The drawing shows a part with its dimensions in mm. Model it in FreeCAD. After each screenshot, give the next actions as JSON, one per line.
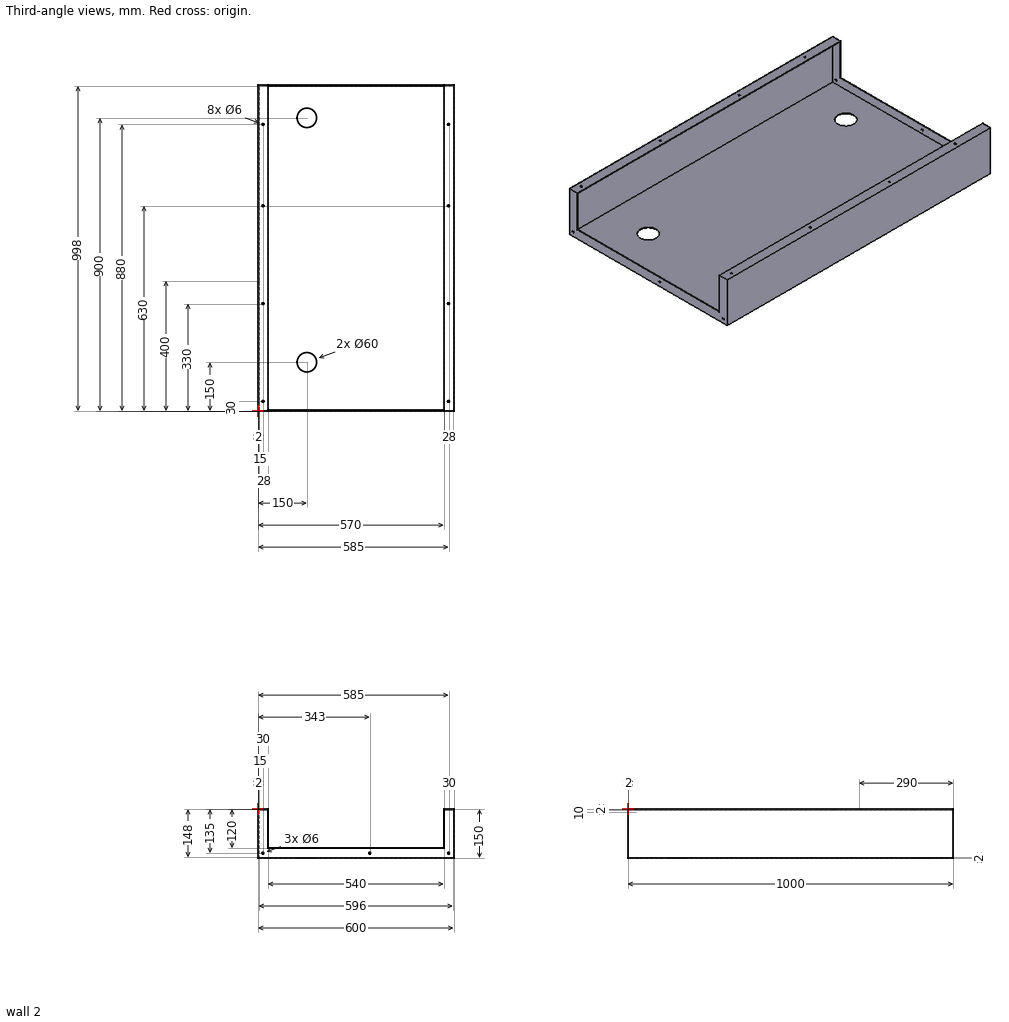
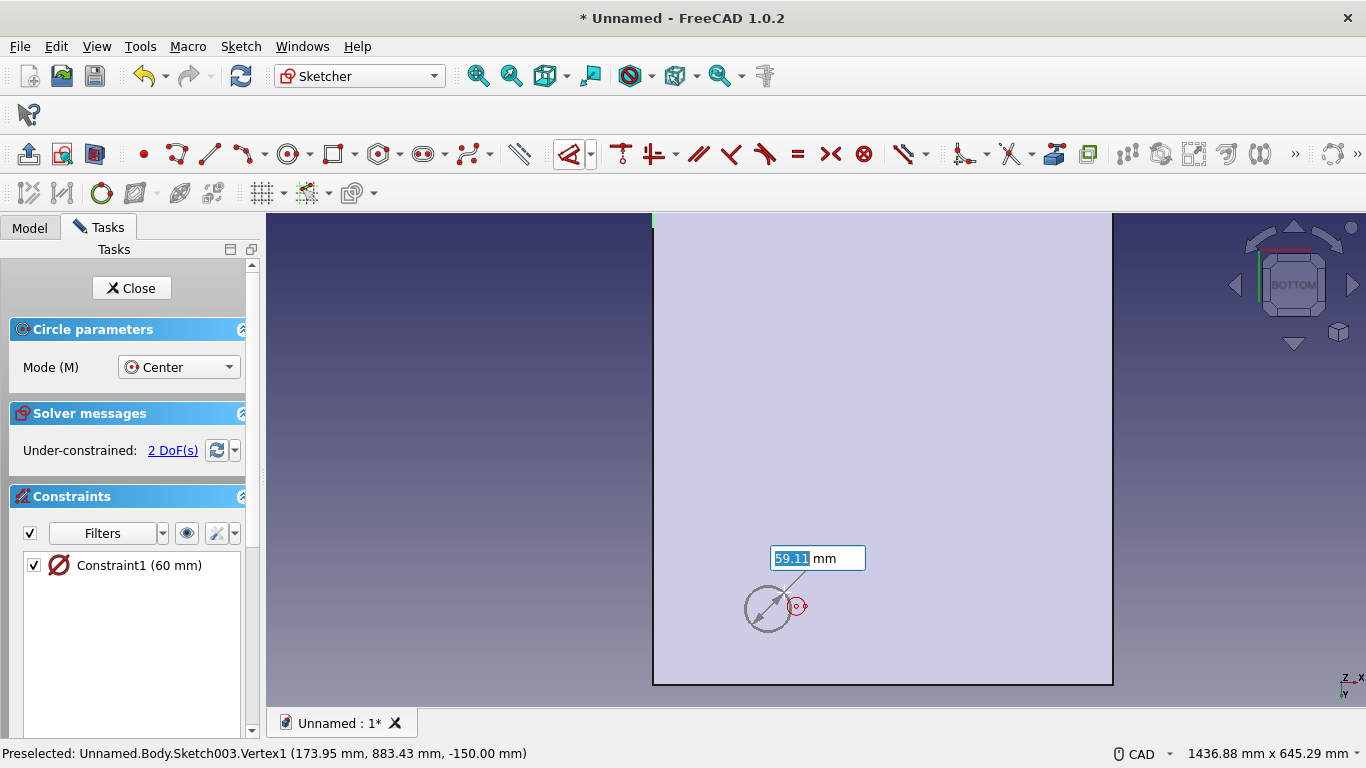
{"action": "type", "text": "60"}
{"action": "key", "text": "Return"}
{"action": "key", "text": "Escape"}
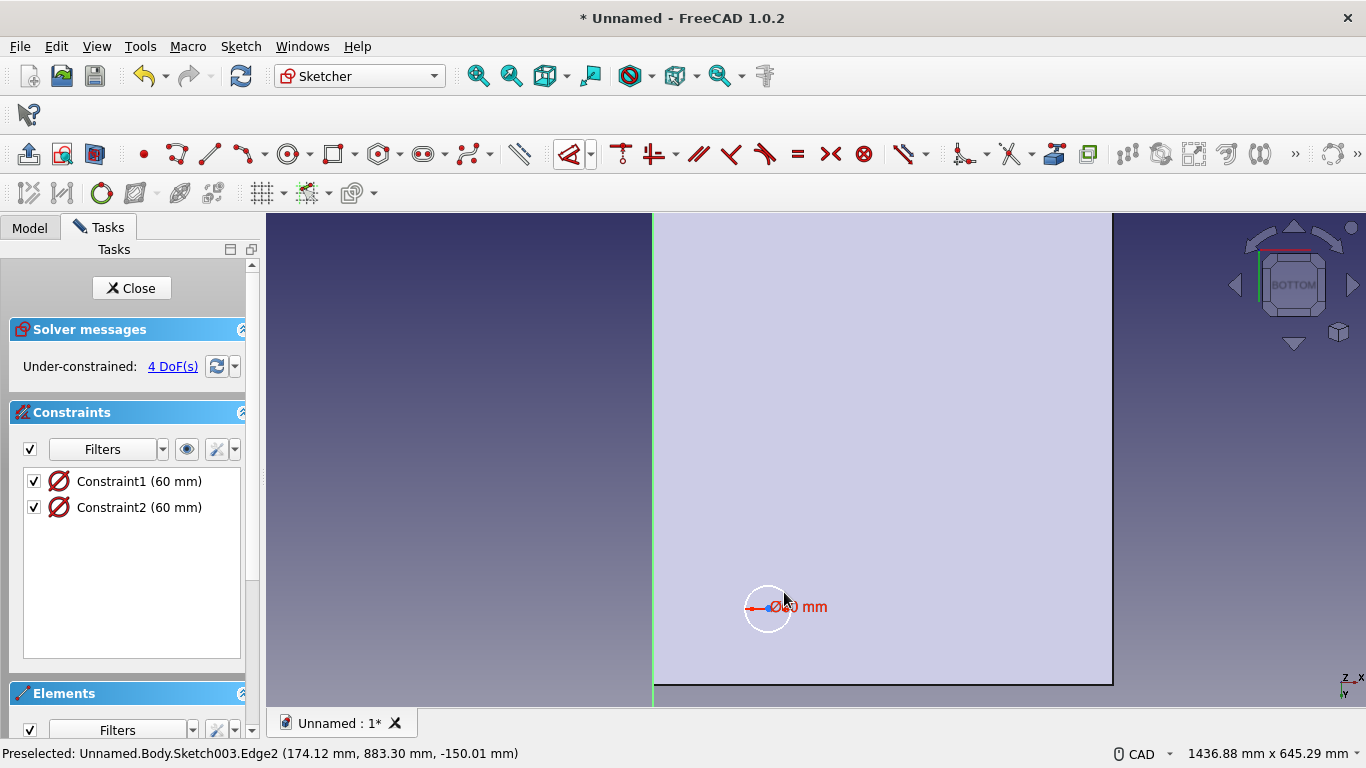
{"action": "scroll", "coordinate": [768, 611], "scroll_direction": "down", "scroll_amount": 4}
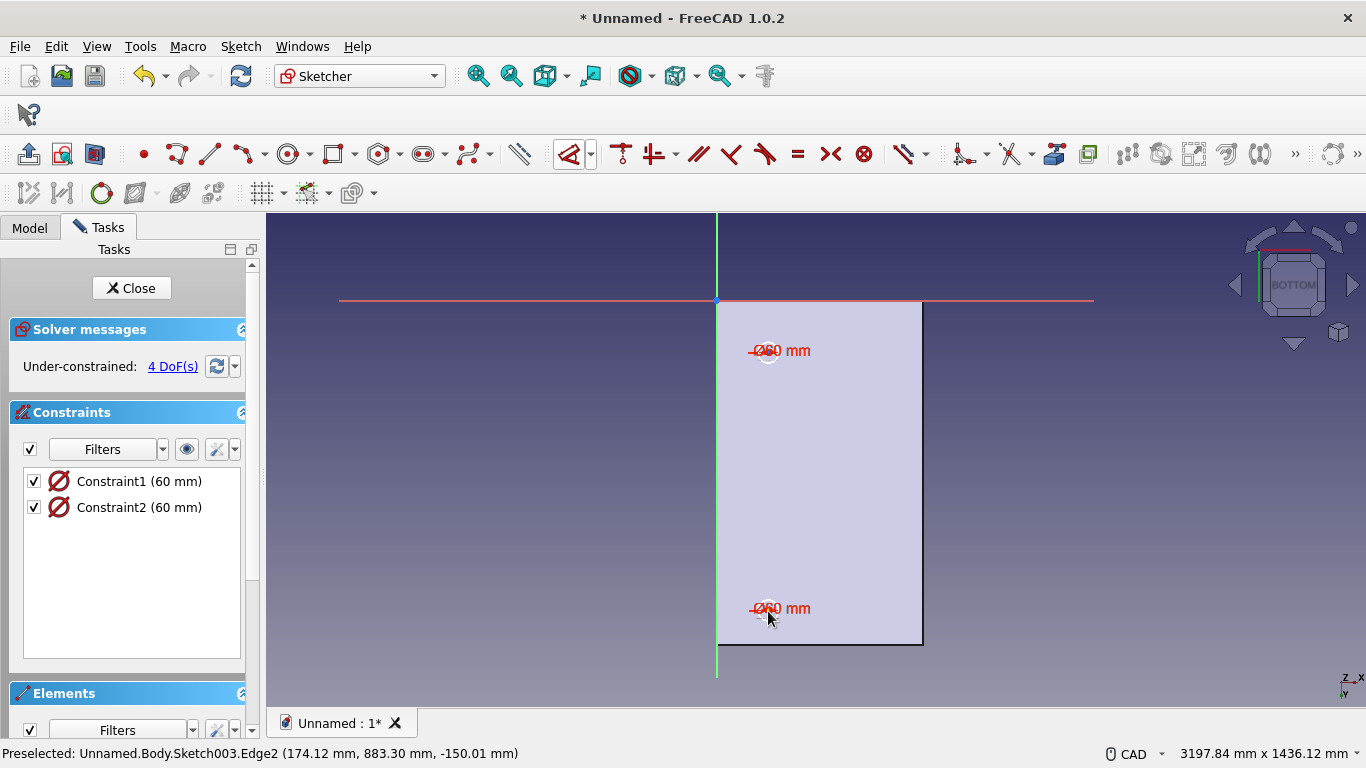
{"action": "left_click", "coordinate": [768, 353]}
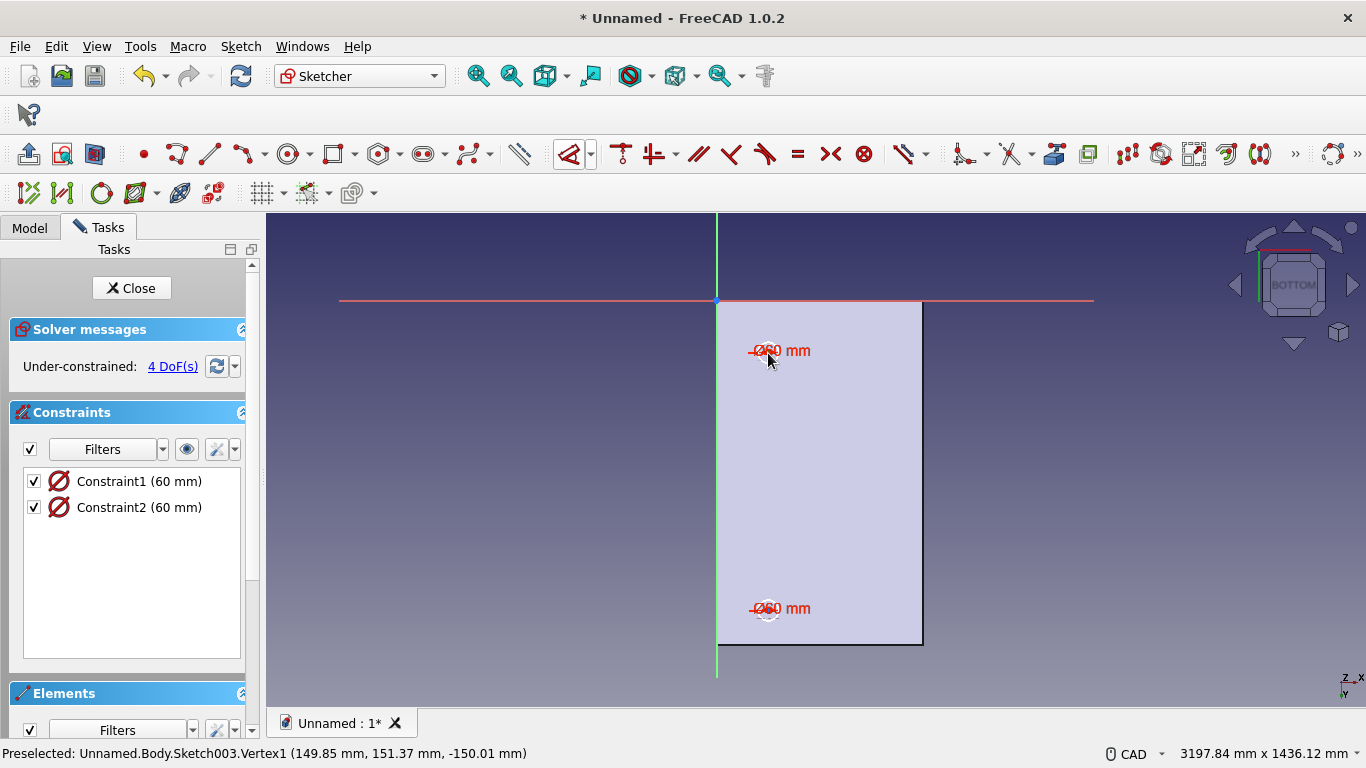
{"action": "left_click", "coordinate": [590, 154]}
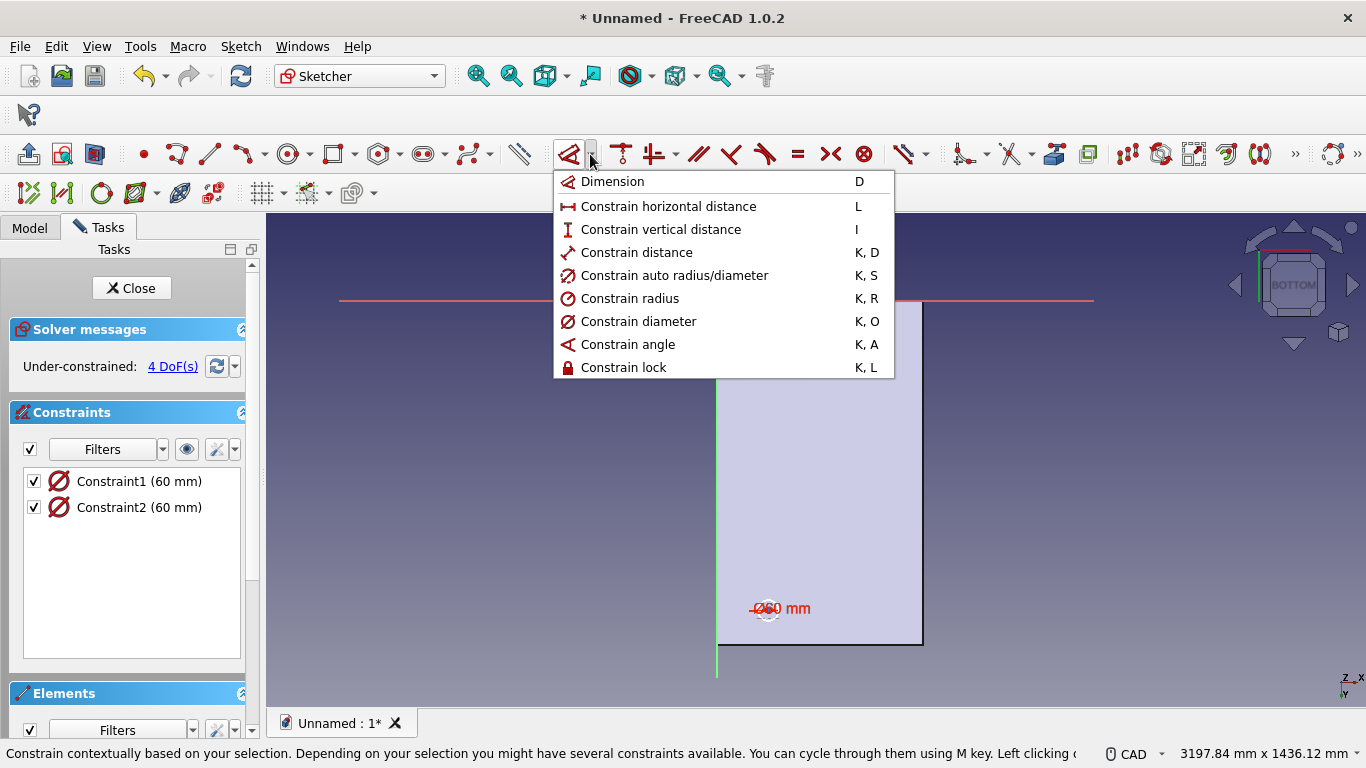
{"action": "left_click", "coordinate": [724, 206]}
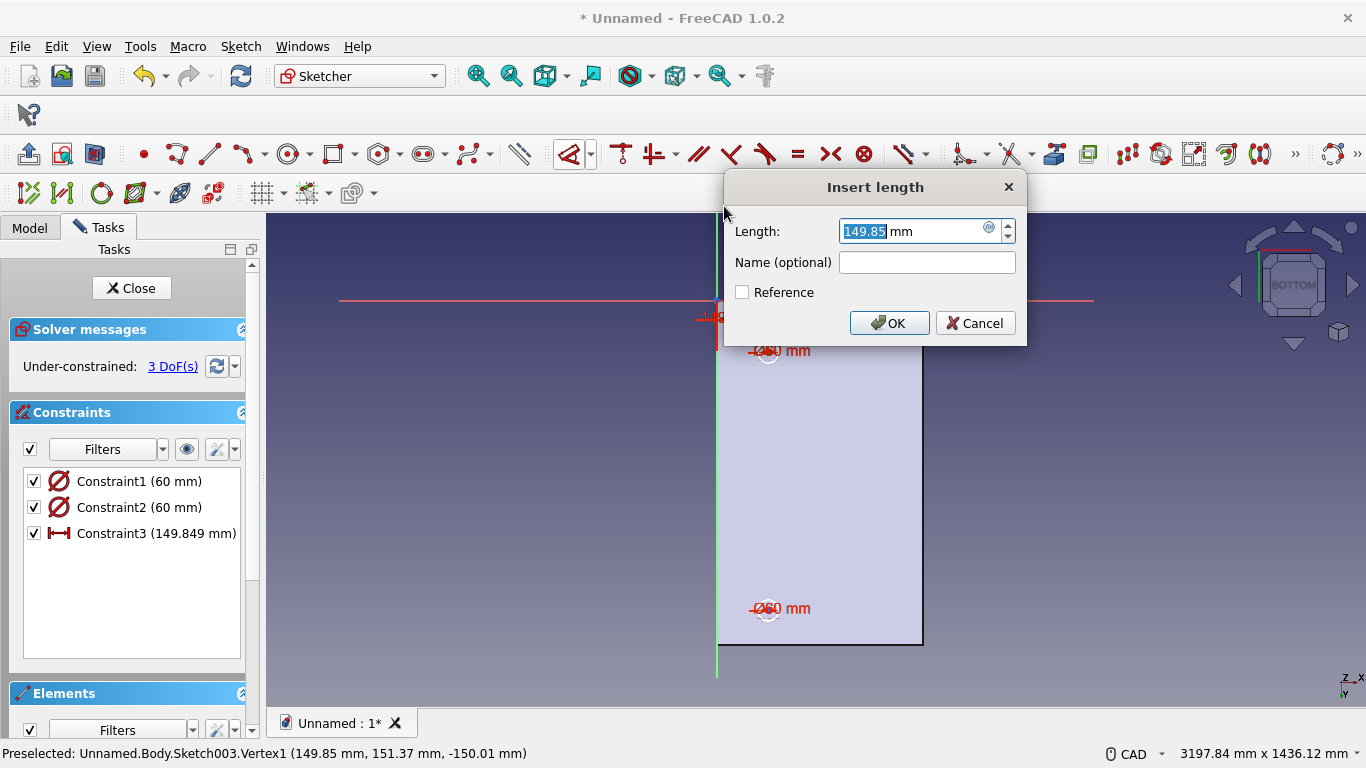
{"action": "type", "text": "150"}
{"action": "key", "text": "Return"}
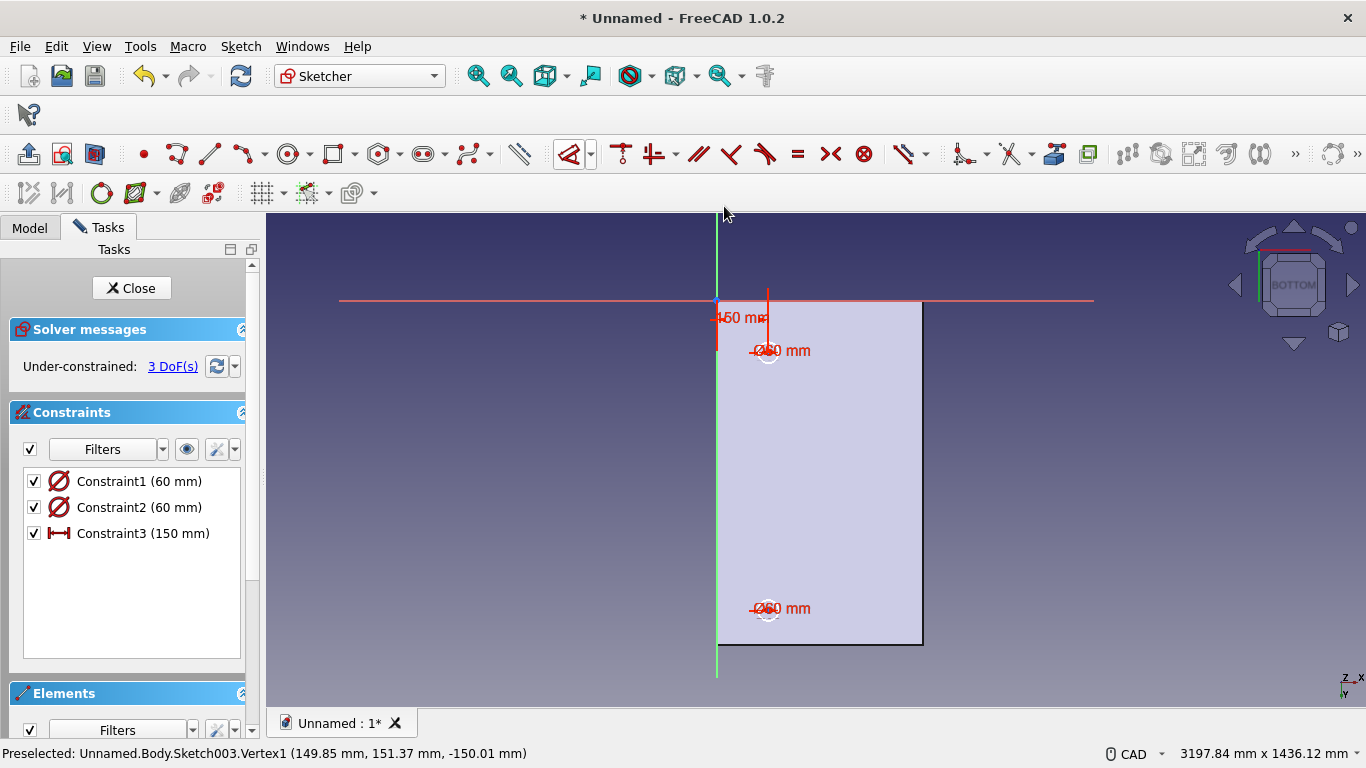
{"action": "left_click", "coordinate": [768, 353]}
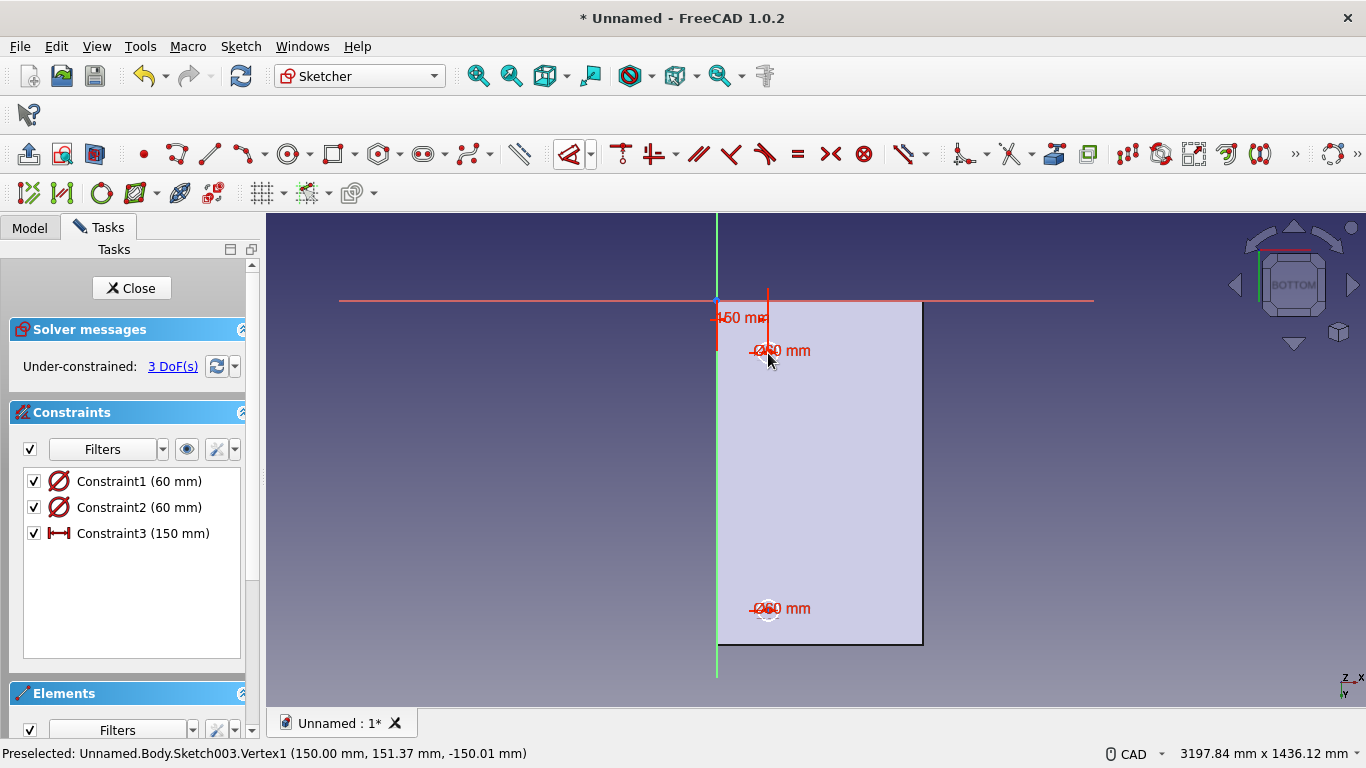
{"action": "key", "text": "i"}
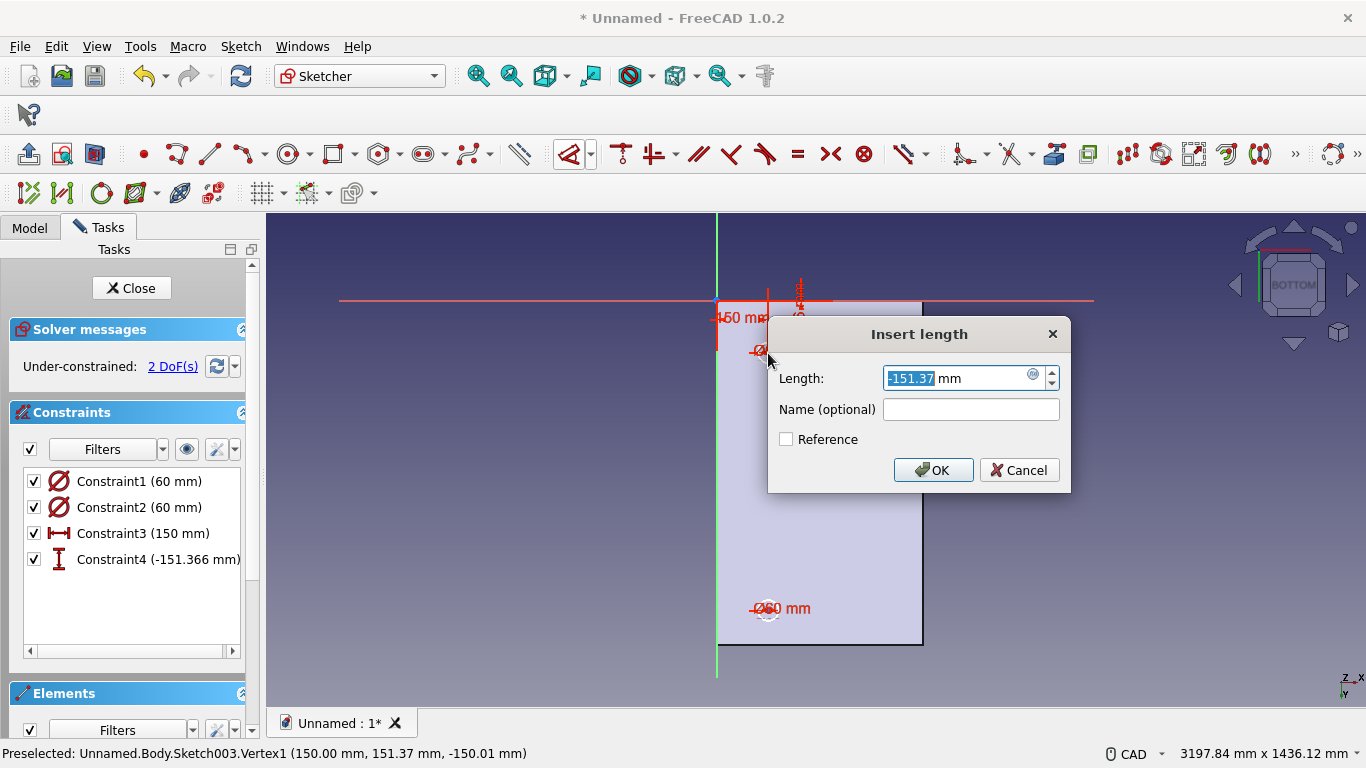
{"action": "type", "text": "-150"}
{"action": "key", "text": "Return"}